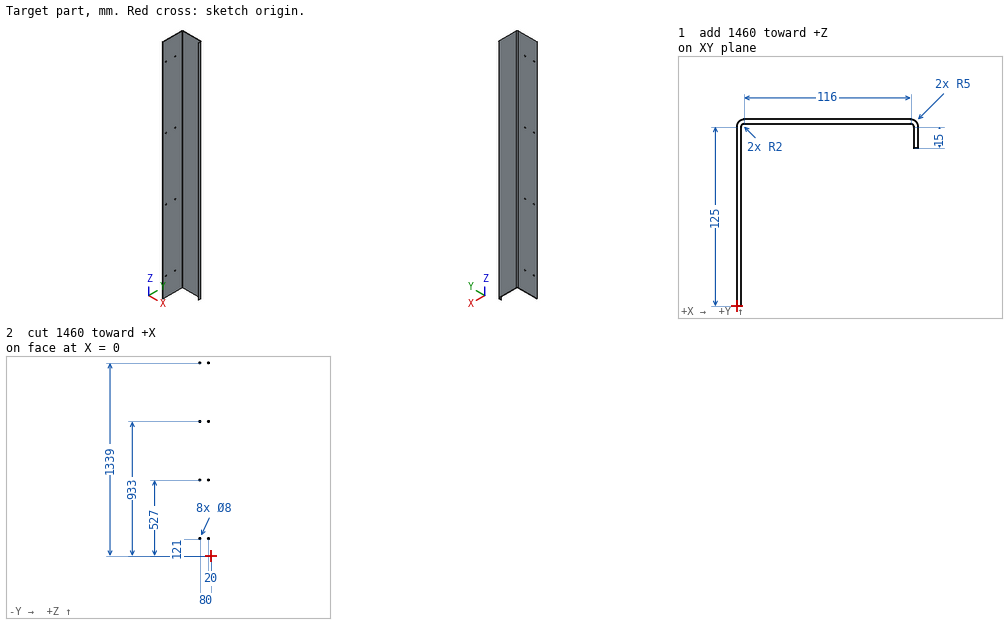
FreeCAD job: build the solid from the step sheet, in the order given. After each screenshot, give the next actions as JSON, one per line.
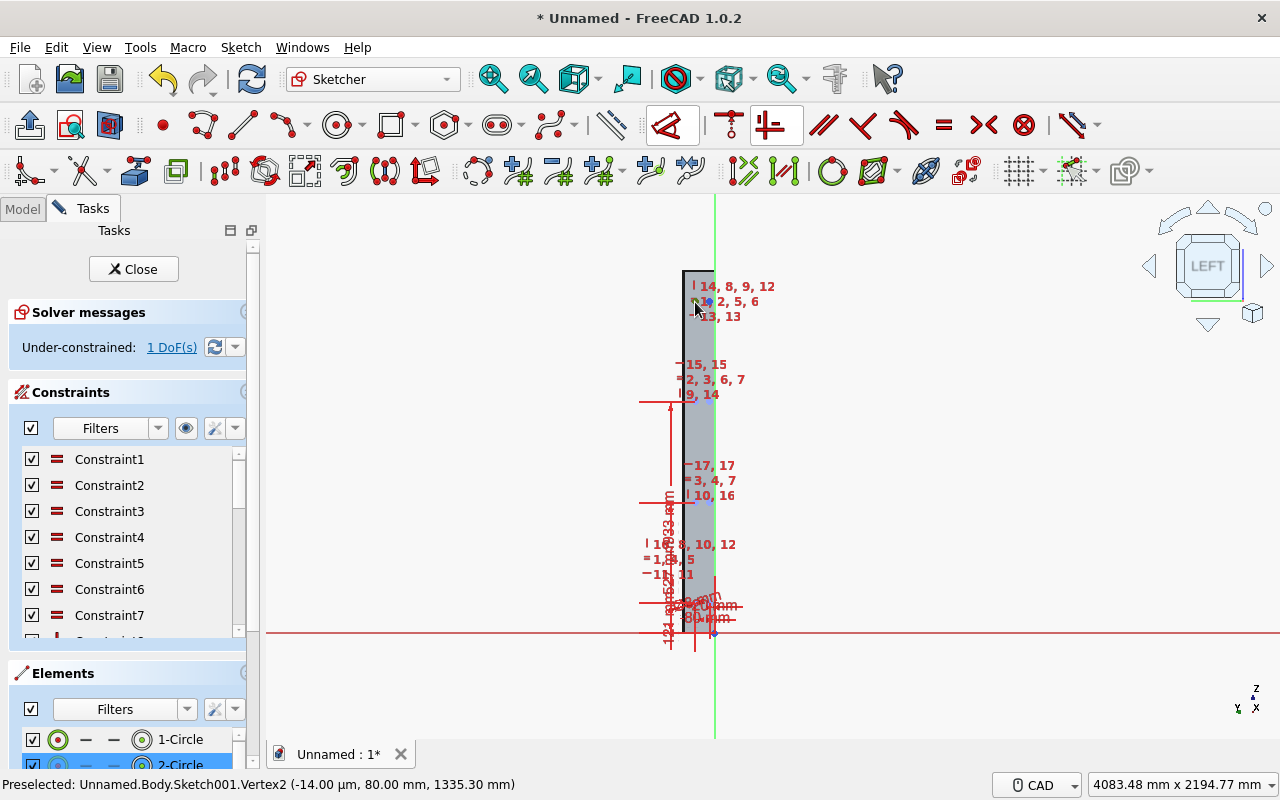
{"action": "left_click", "coordinate": [694, 126]}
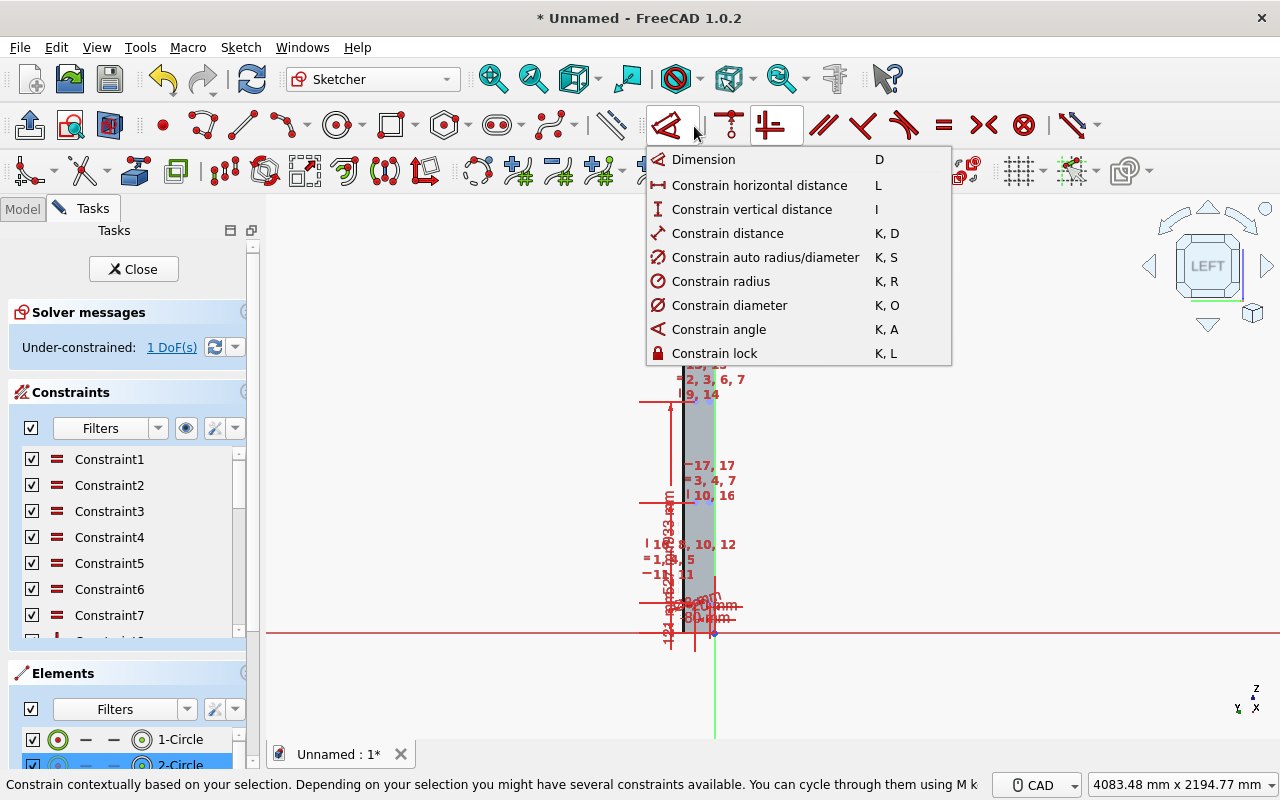
{"action": "left_click", "coordinate": [799, 209]}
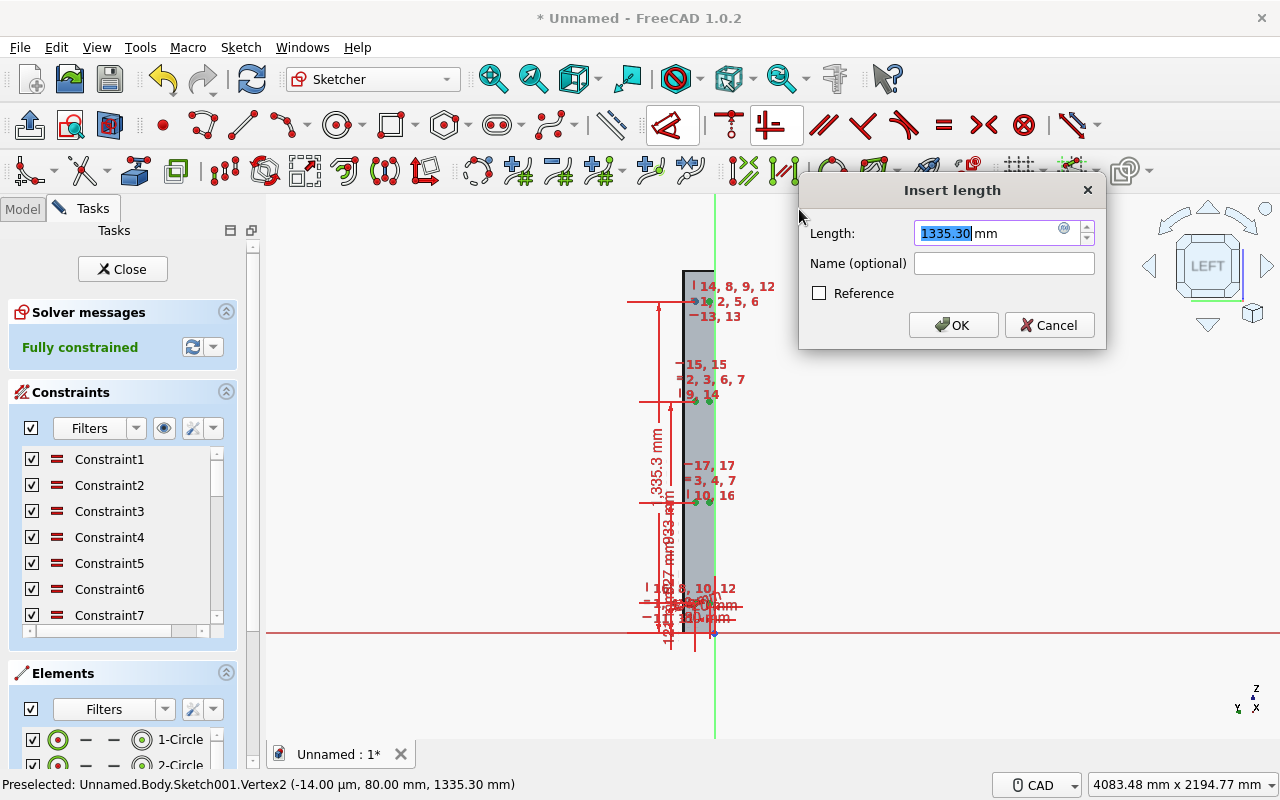
{"action": "type", "text": "1339"}
{"action": "key", "text": "Return"}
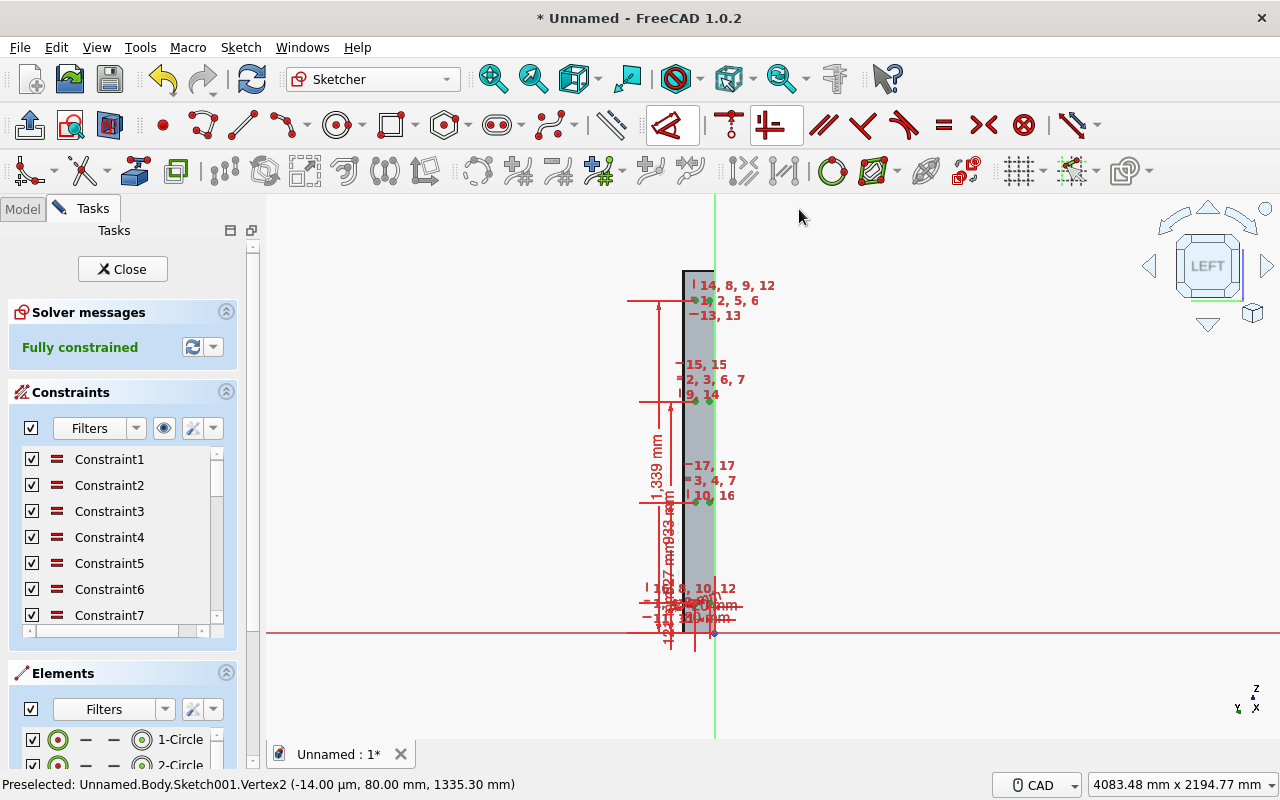
{"action": "left_click", "coordinate": [123, 269]}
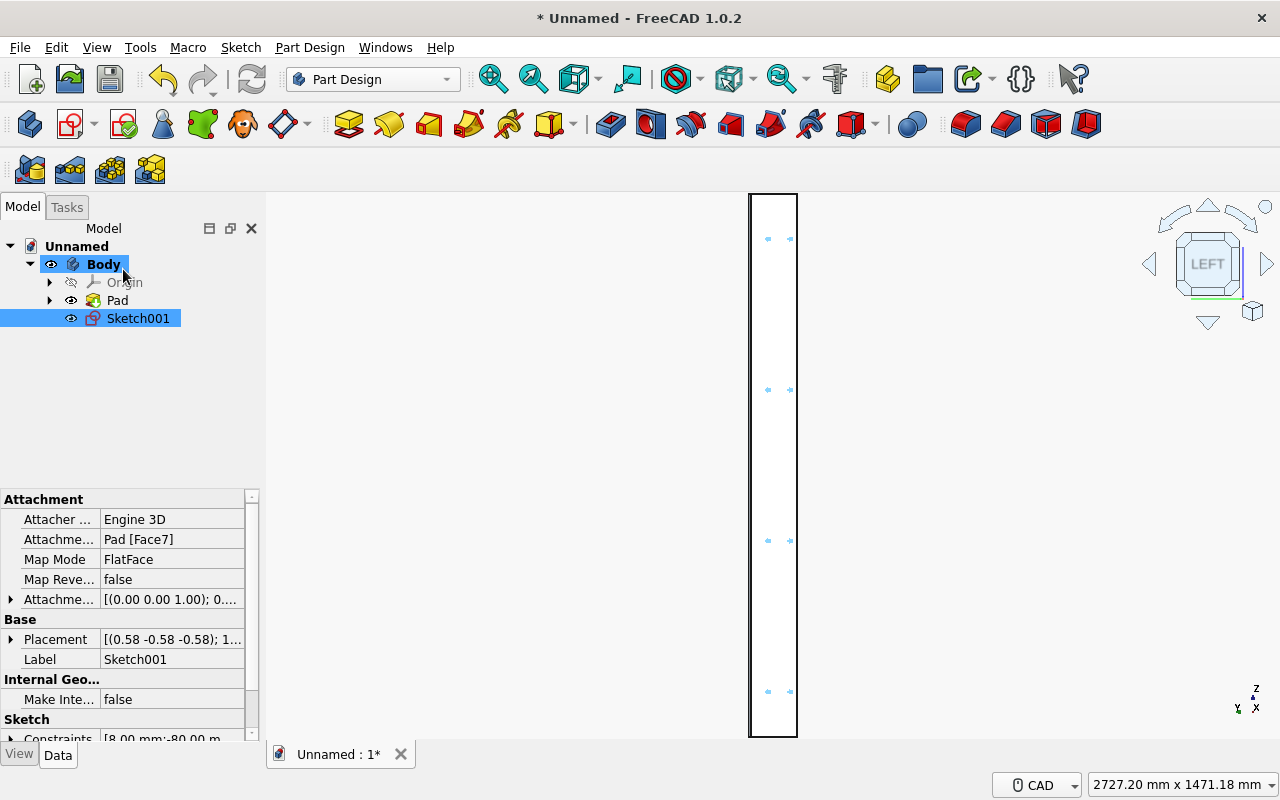
{"action": "left_click", "coordinate": [612, 124]}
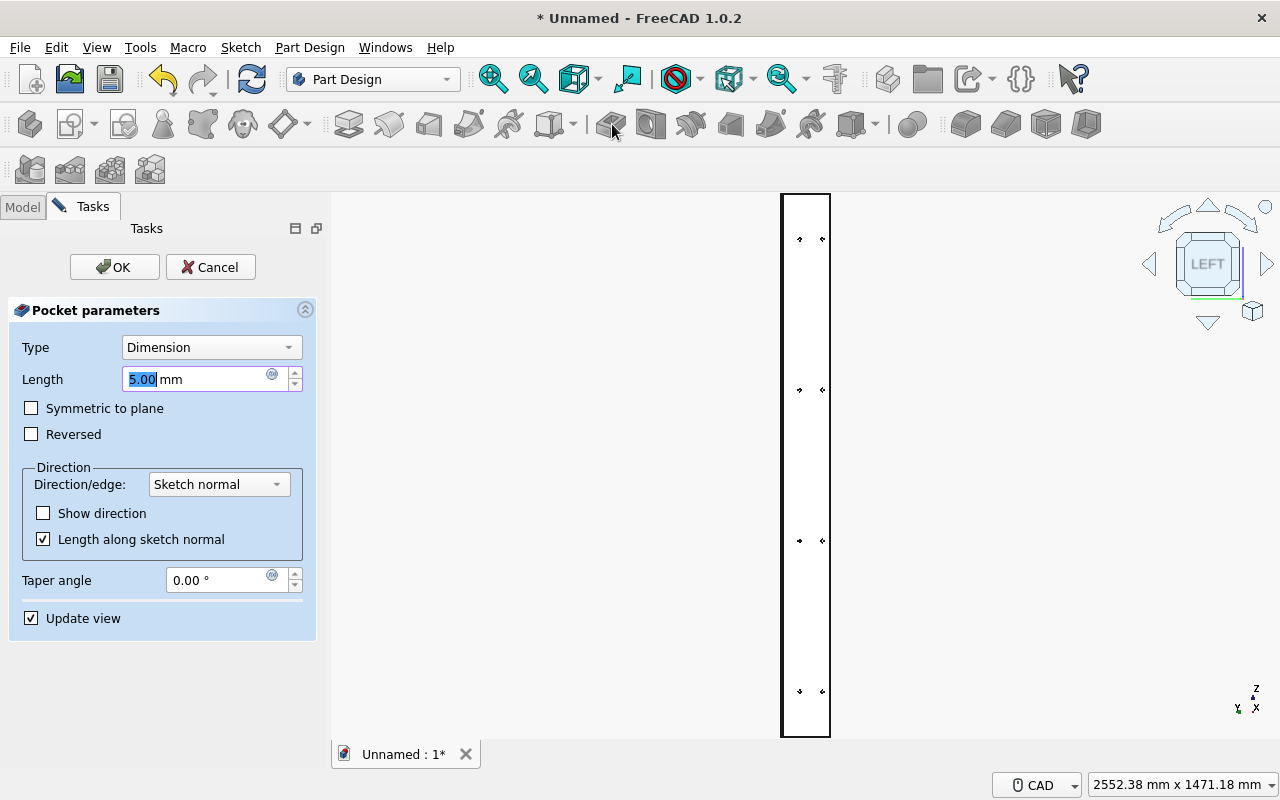
{"action": "type", "text": "1460"}
{"action": "key", "text": "Tab"}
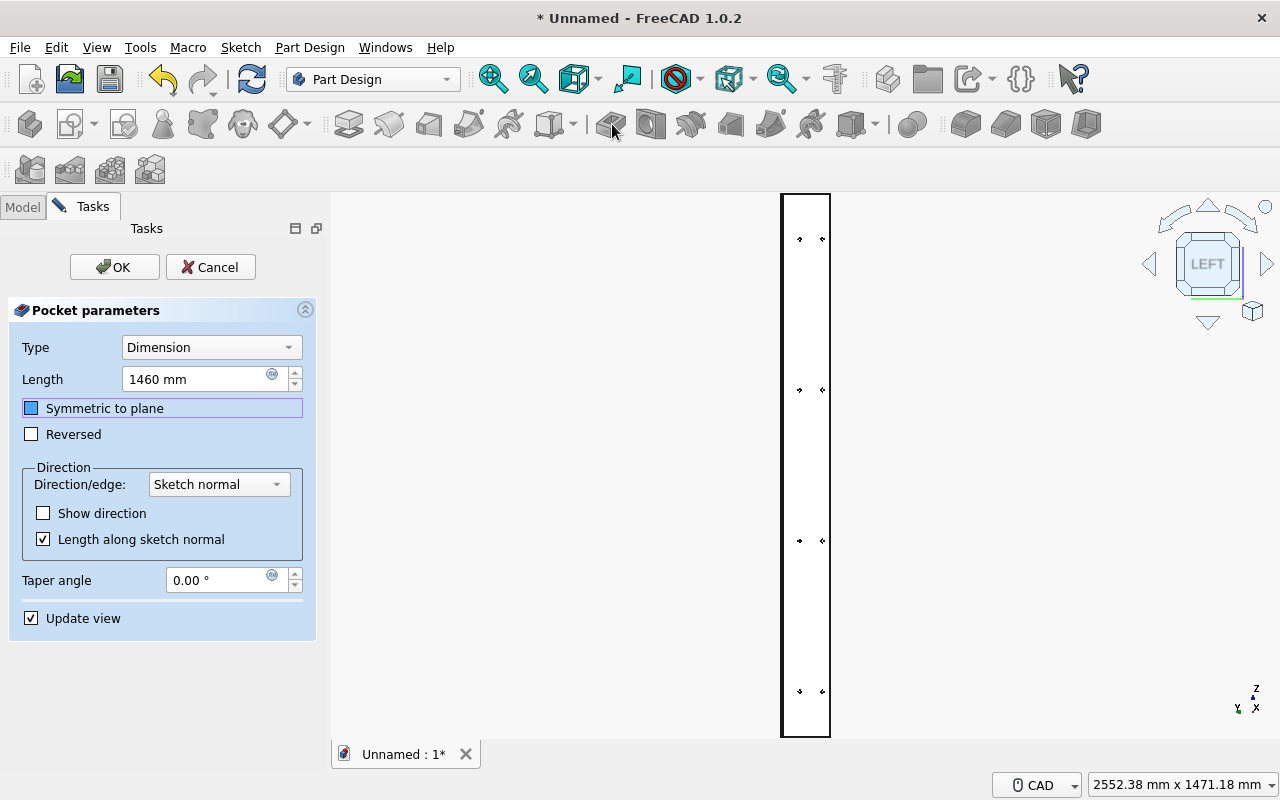
{"action": "left_click", "coordinate": [115, 267]}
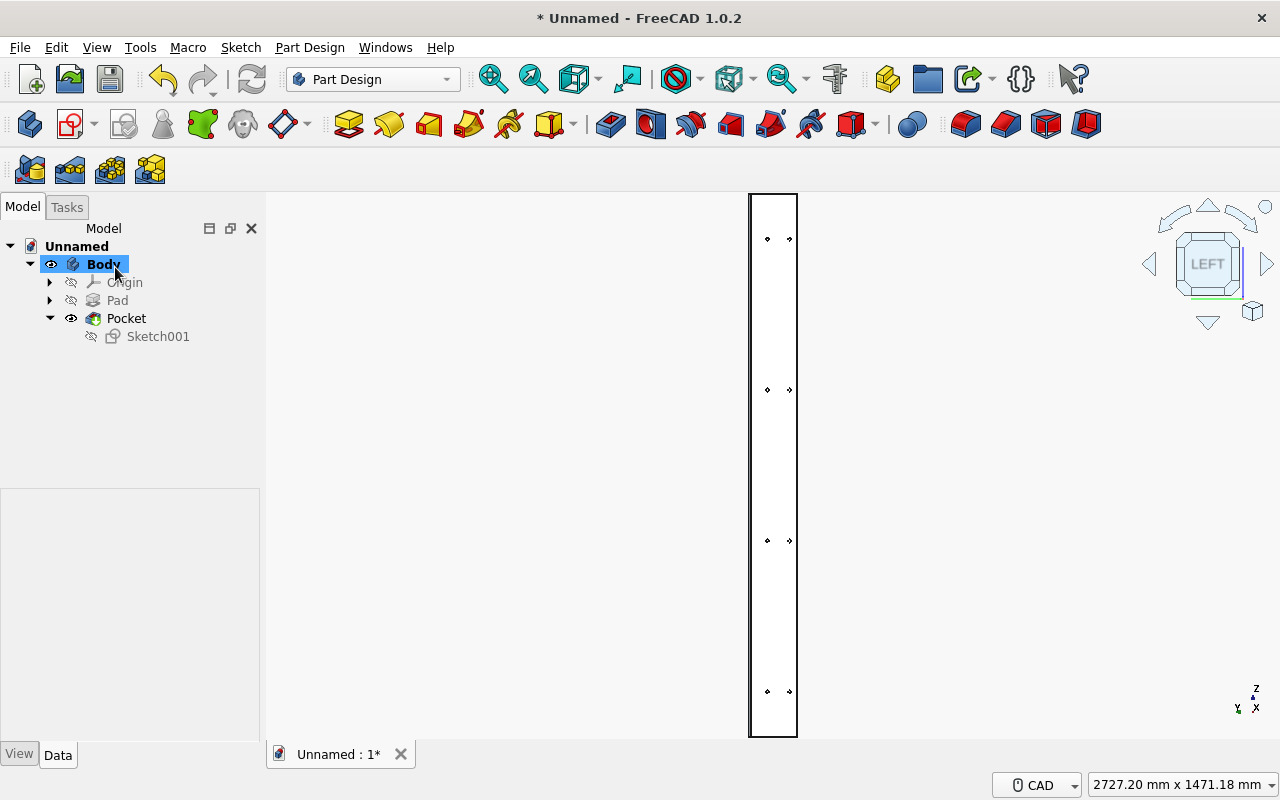
{"action": "key", "text": "0"}